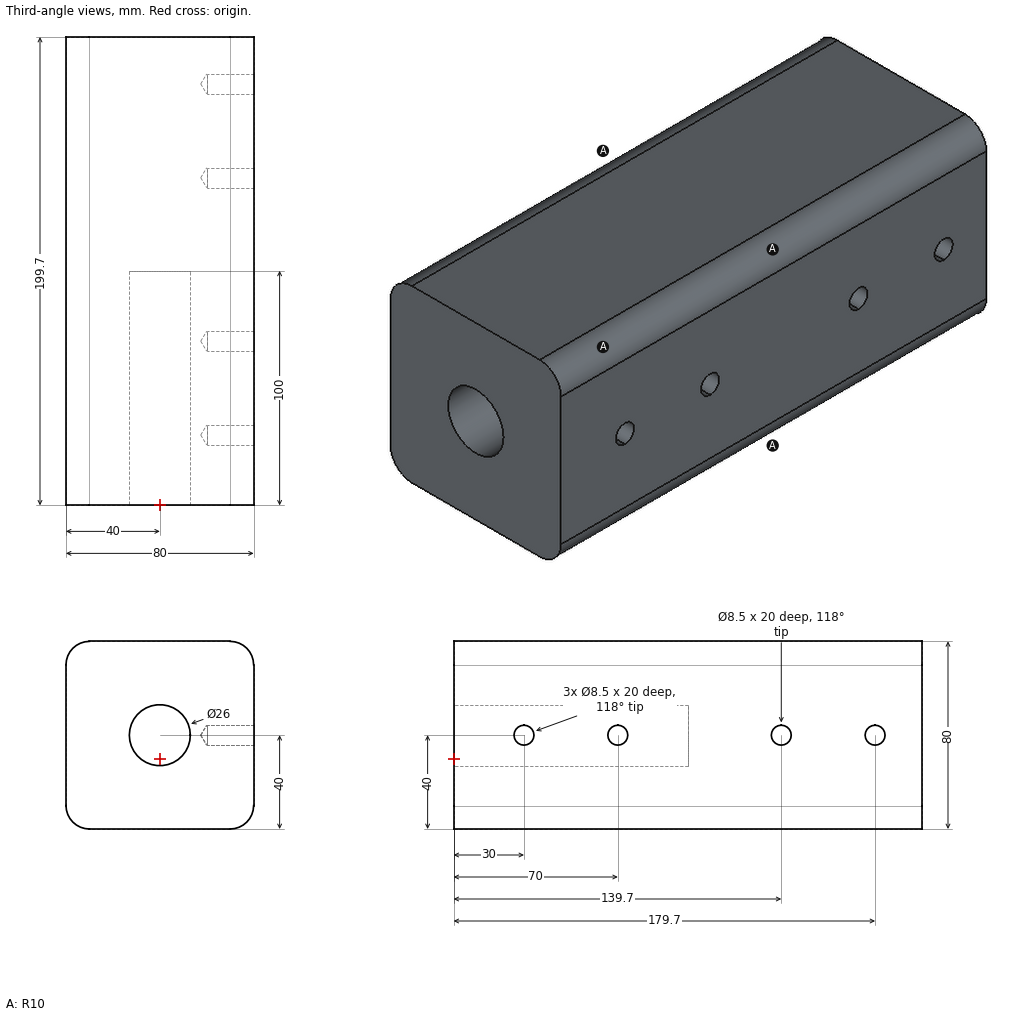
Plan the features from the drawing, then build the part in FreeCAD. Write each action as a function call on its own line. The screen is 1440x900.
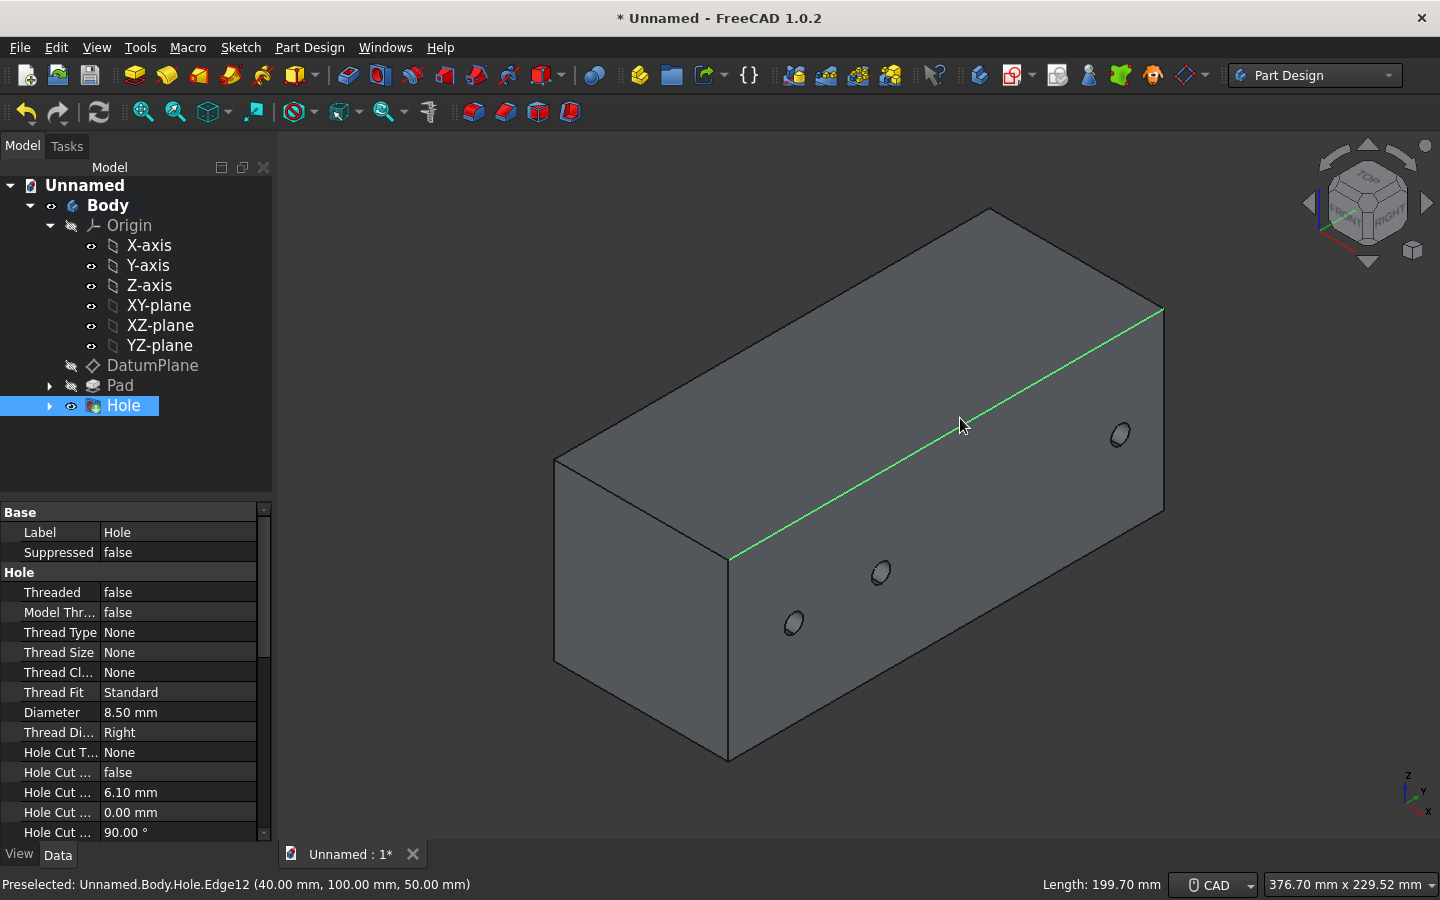
key(2)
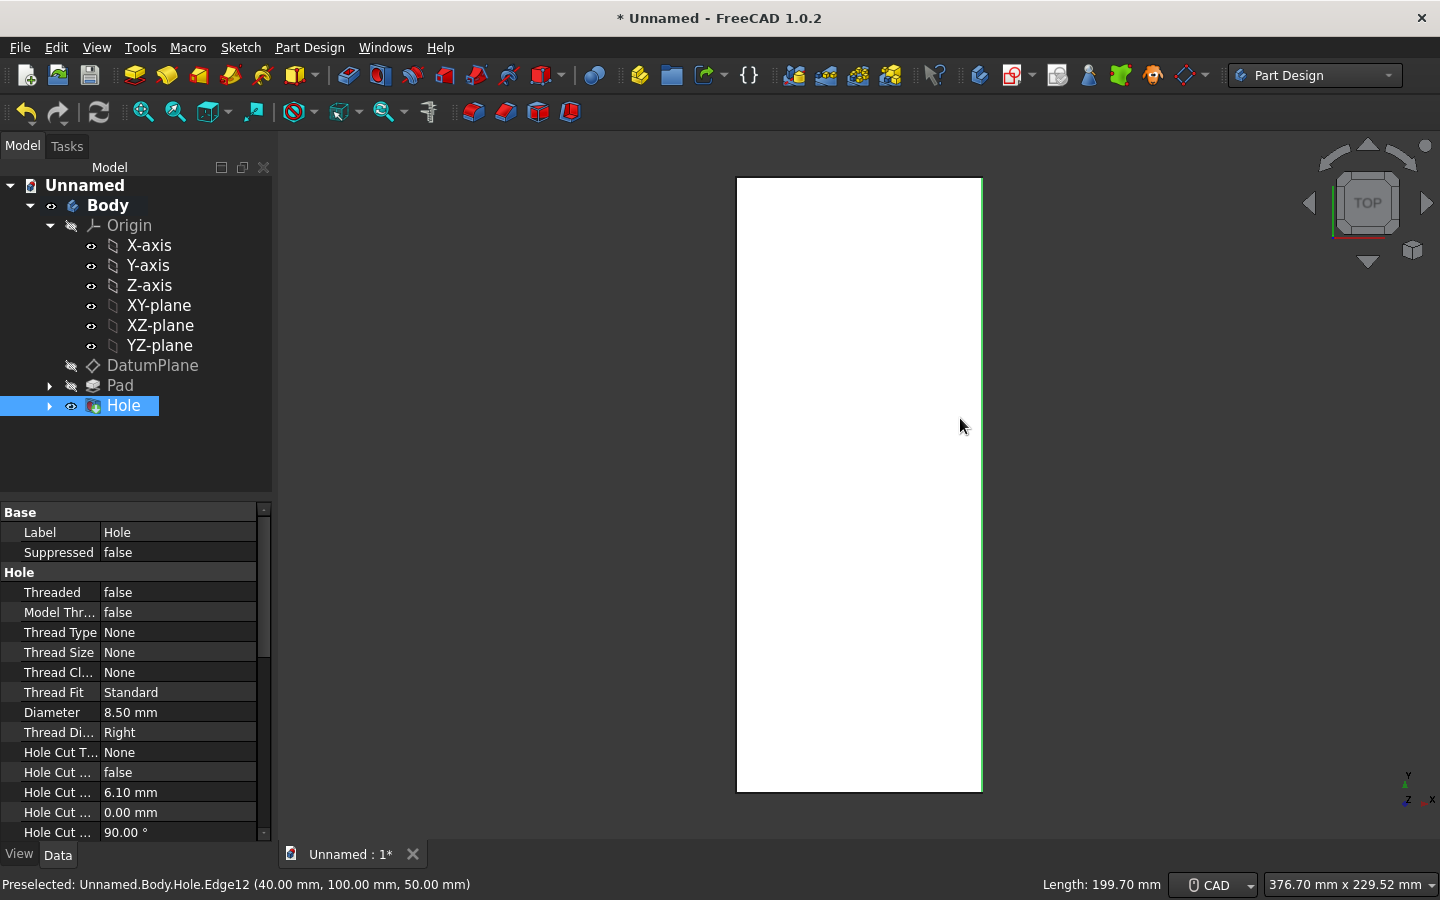
click(736, 484, ctrl)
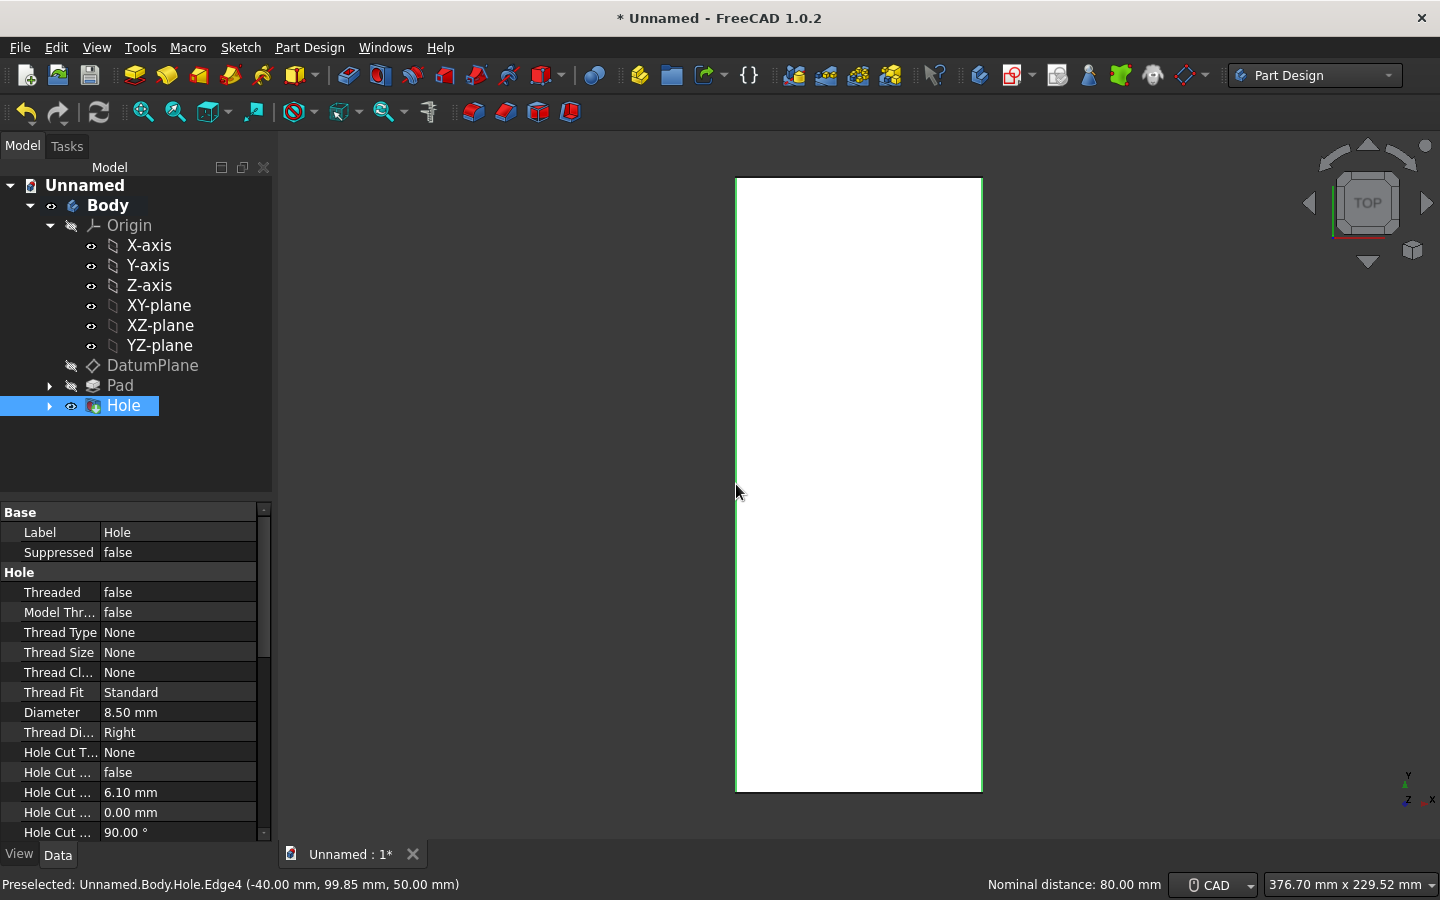
key(1)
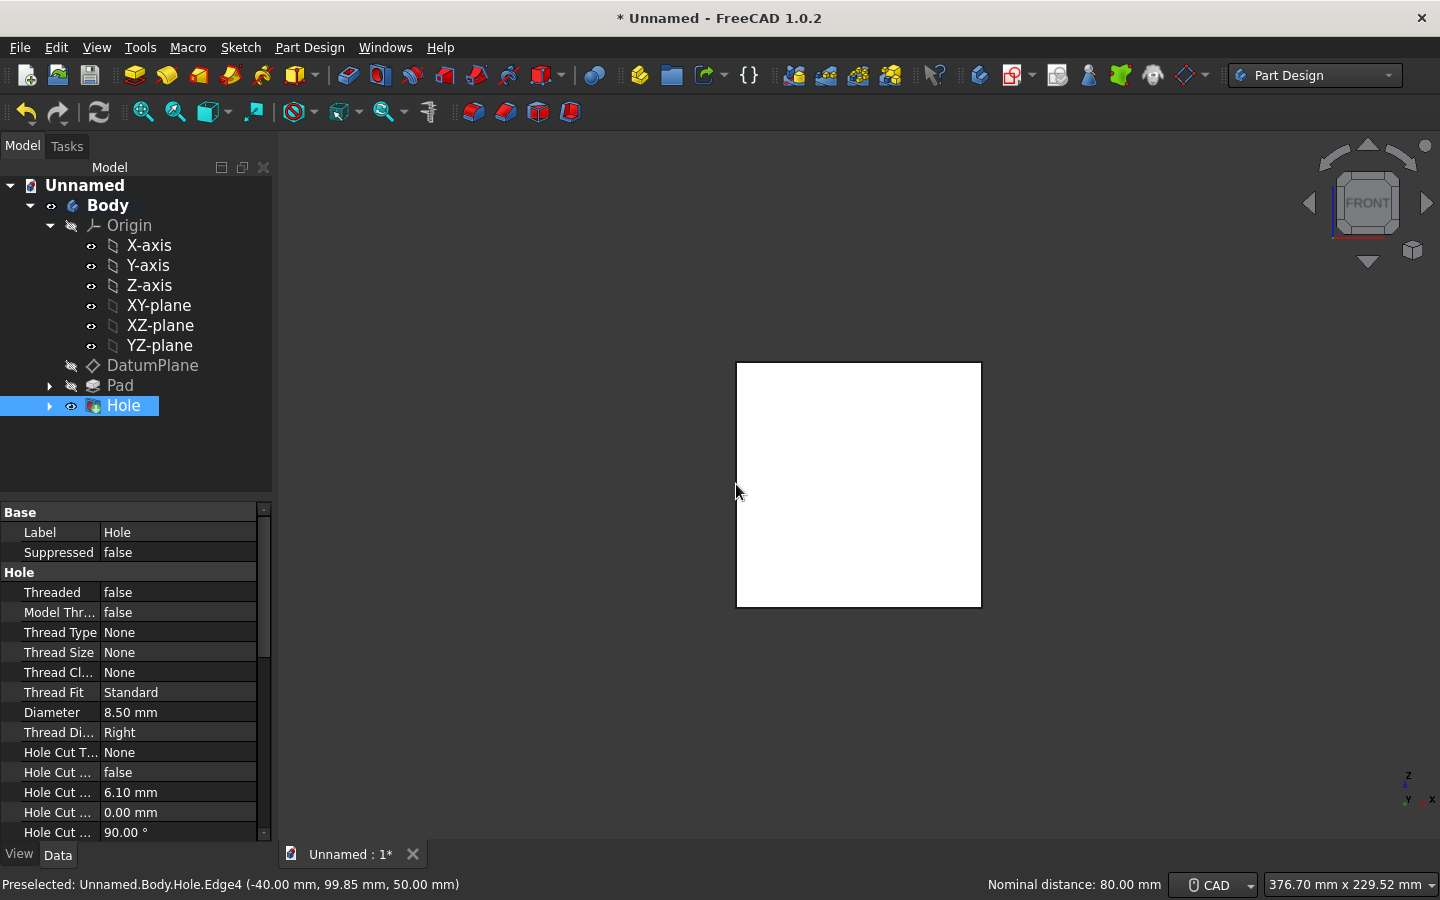
click(144, 112)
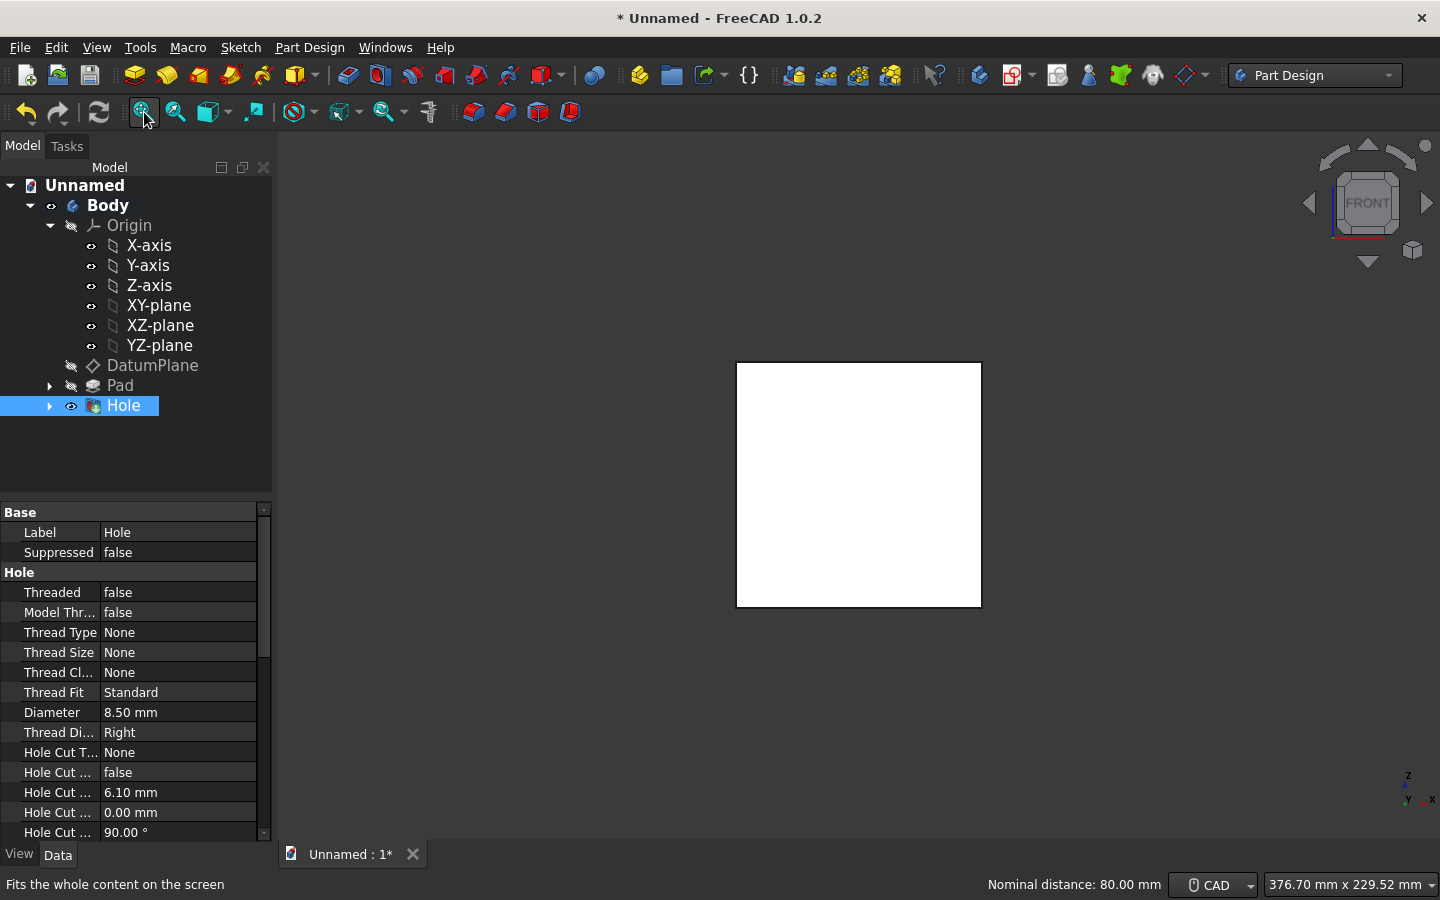
key(3)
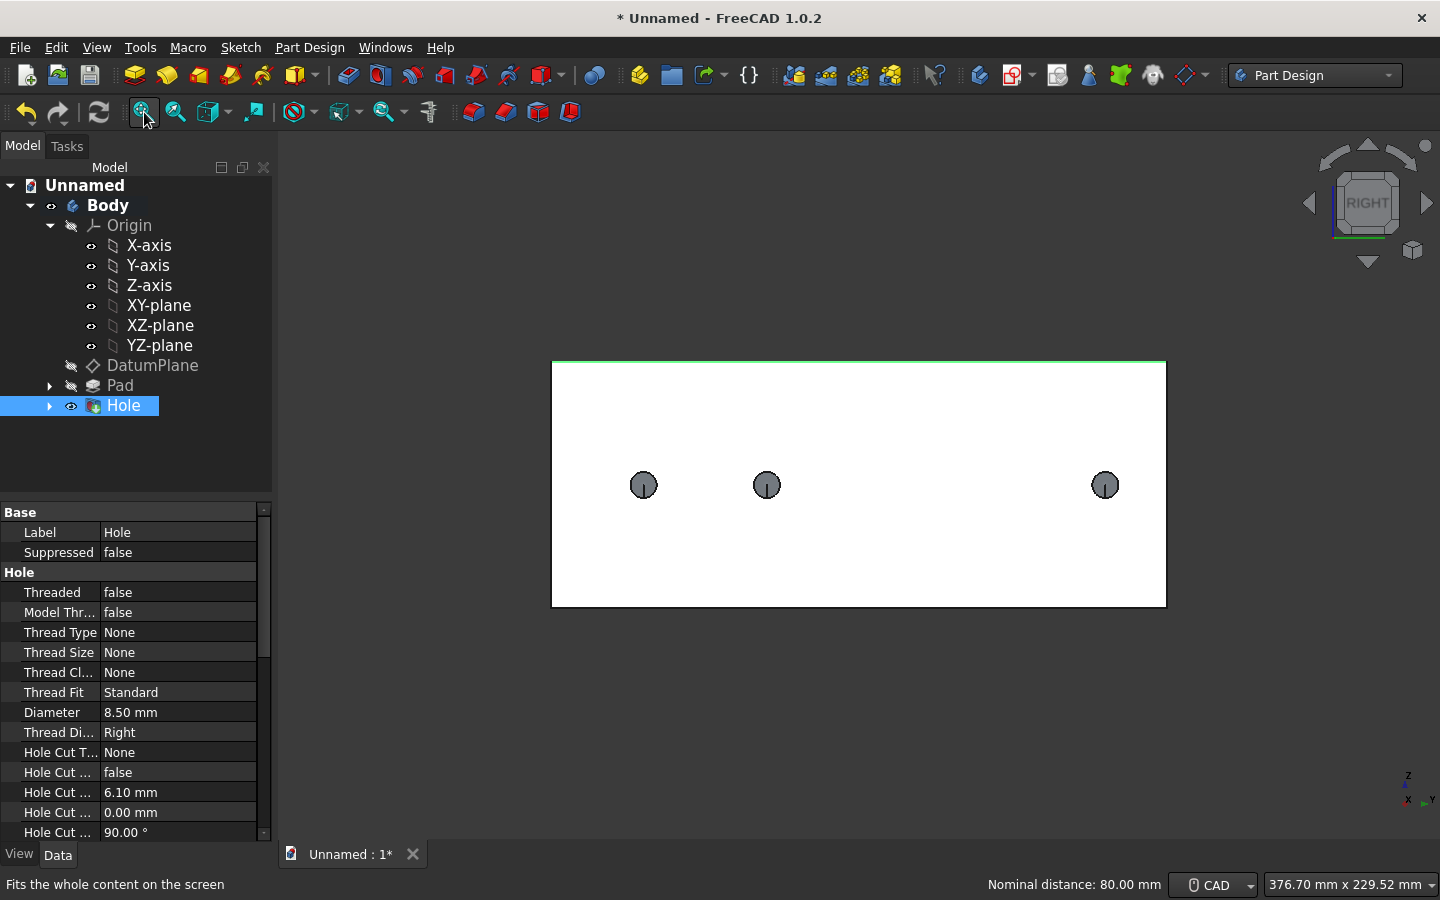
click(859, 607, ctrl)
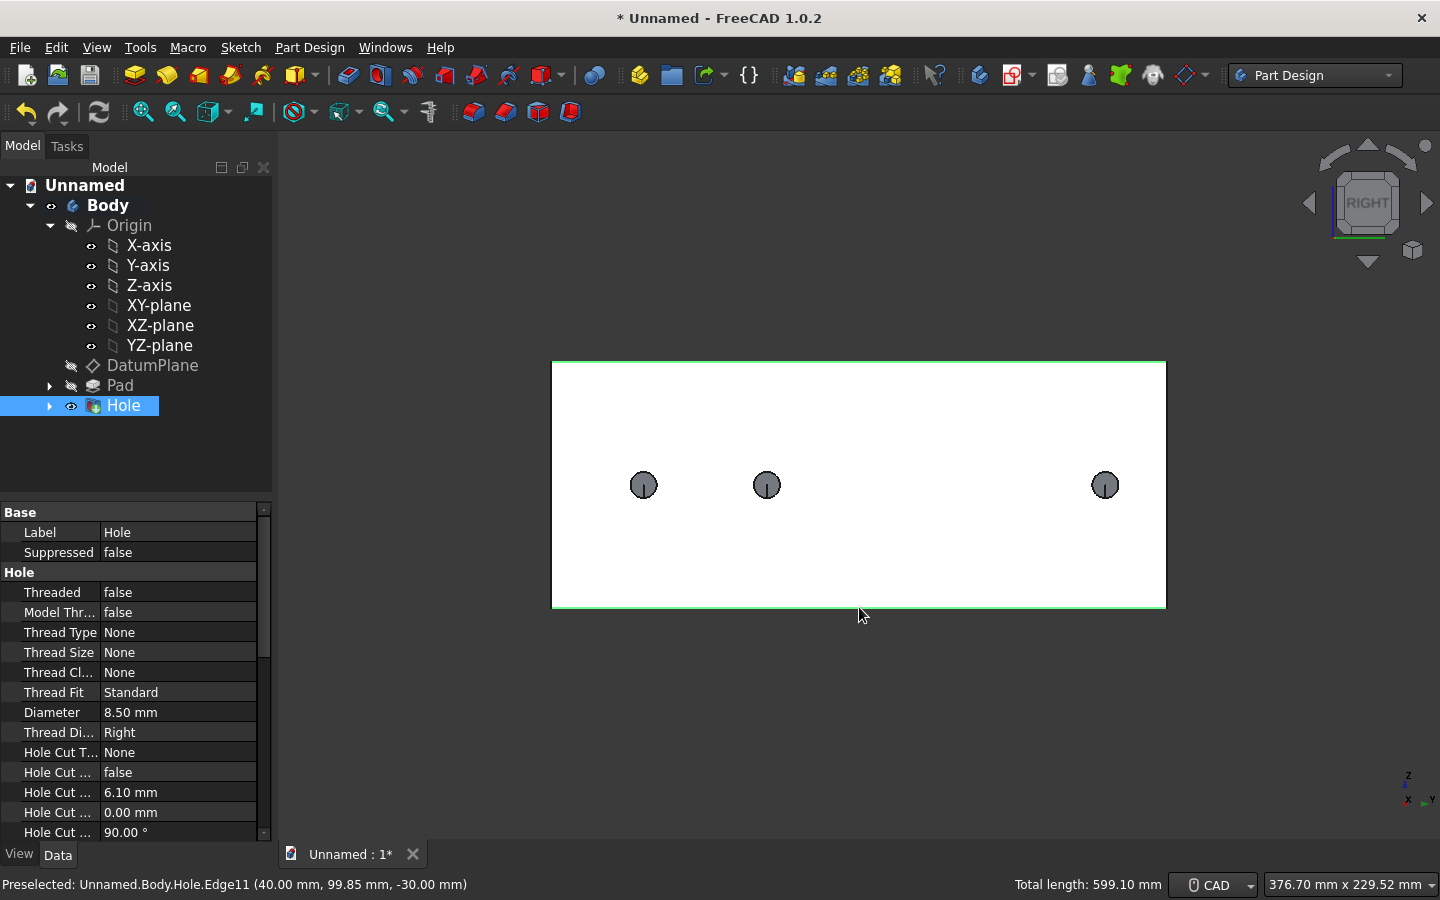
key(5)